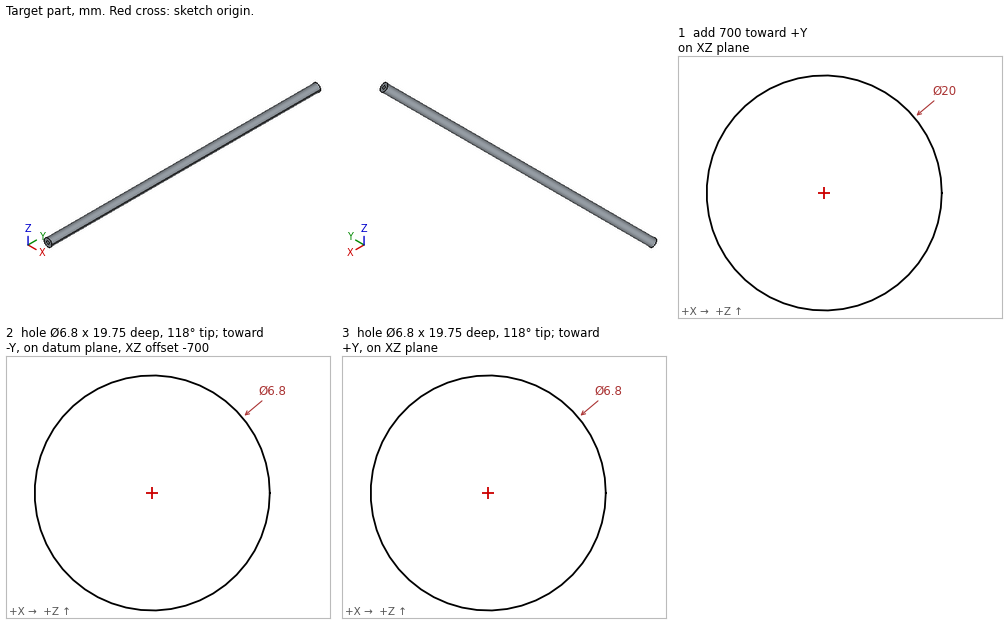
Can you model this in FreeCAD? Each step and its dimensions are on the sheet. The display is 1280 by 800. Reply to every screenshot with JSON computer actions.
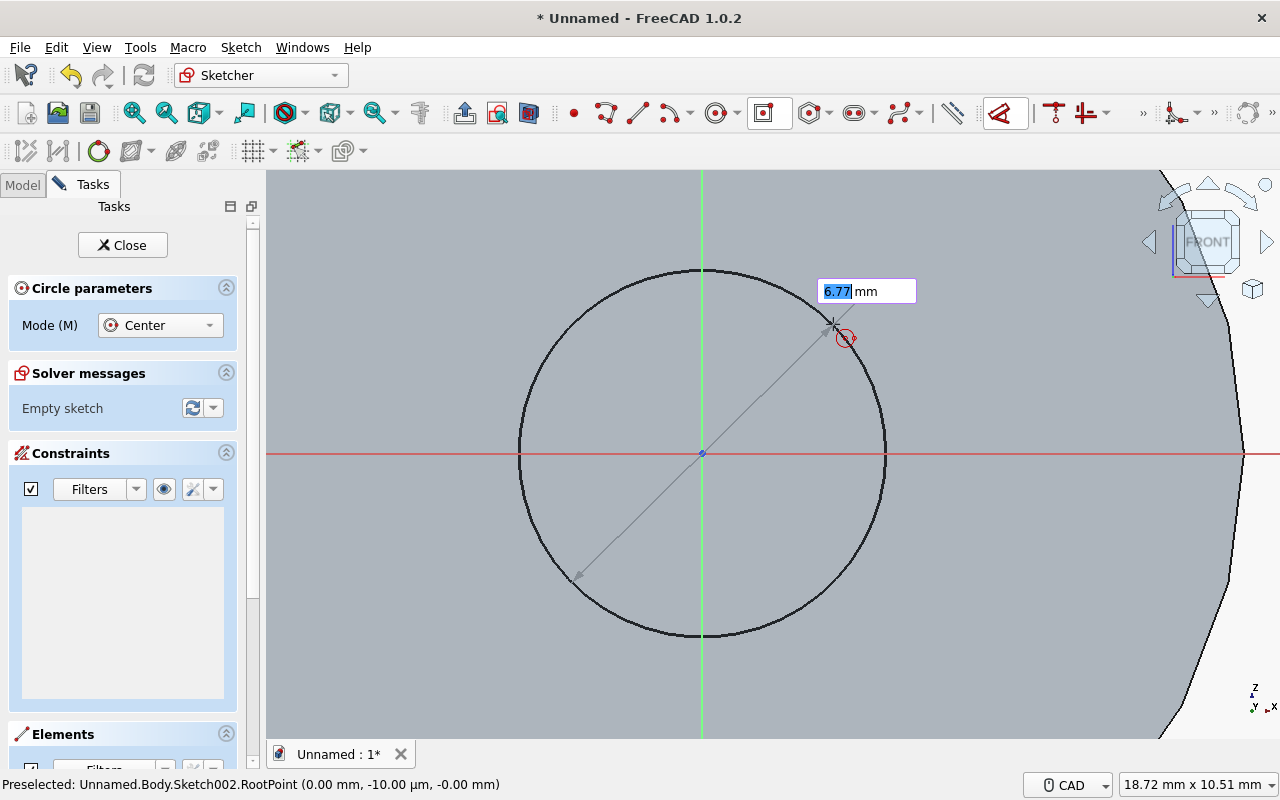
{"action": "type", "text": "6.8"}
{"action": "key", "text": "Return"}
{"action": "key", "text": "Escape"}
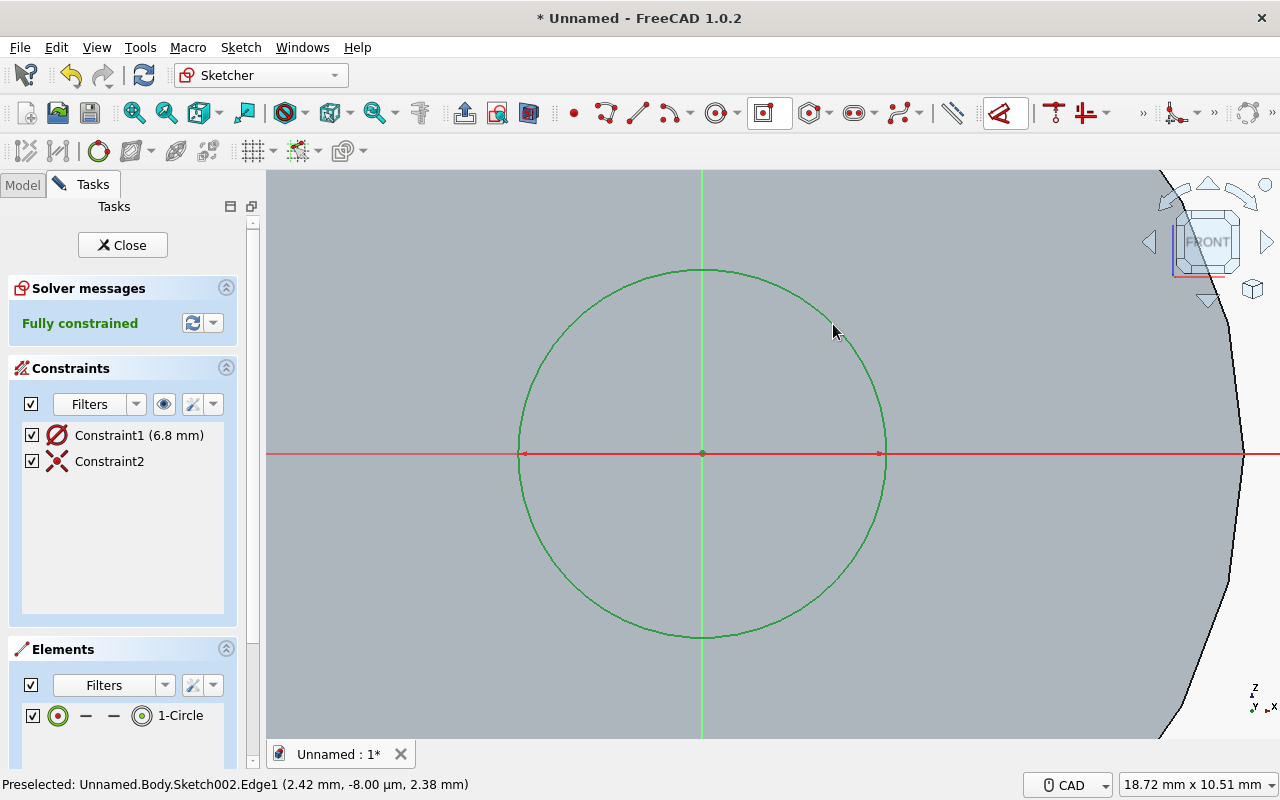
{"action": "left_click", "coordinate": [123, 245]}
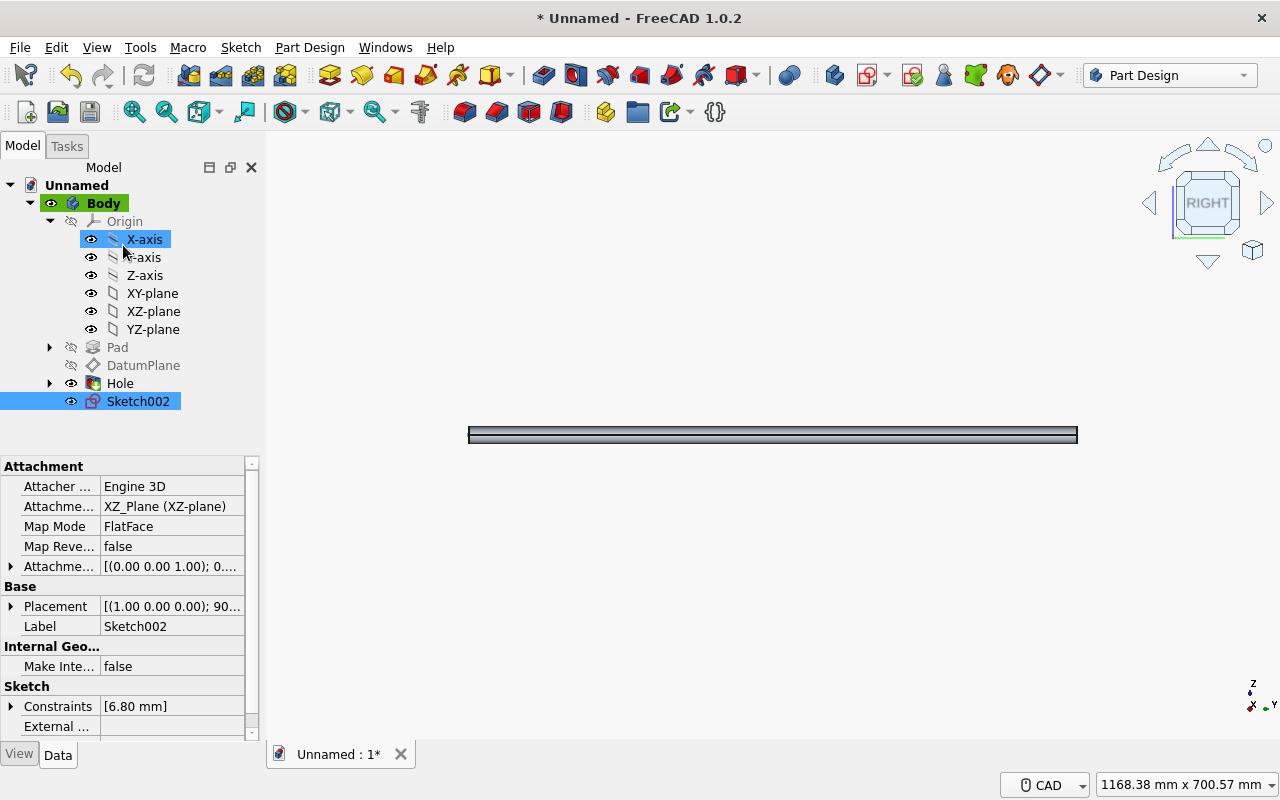
{"action": "left_click", "coordinate": [576, 76]}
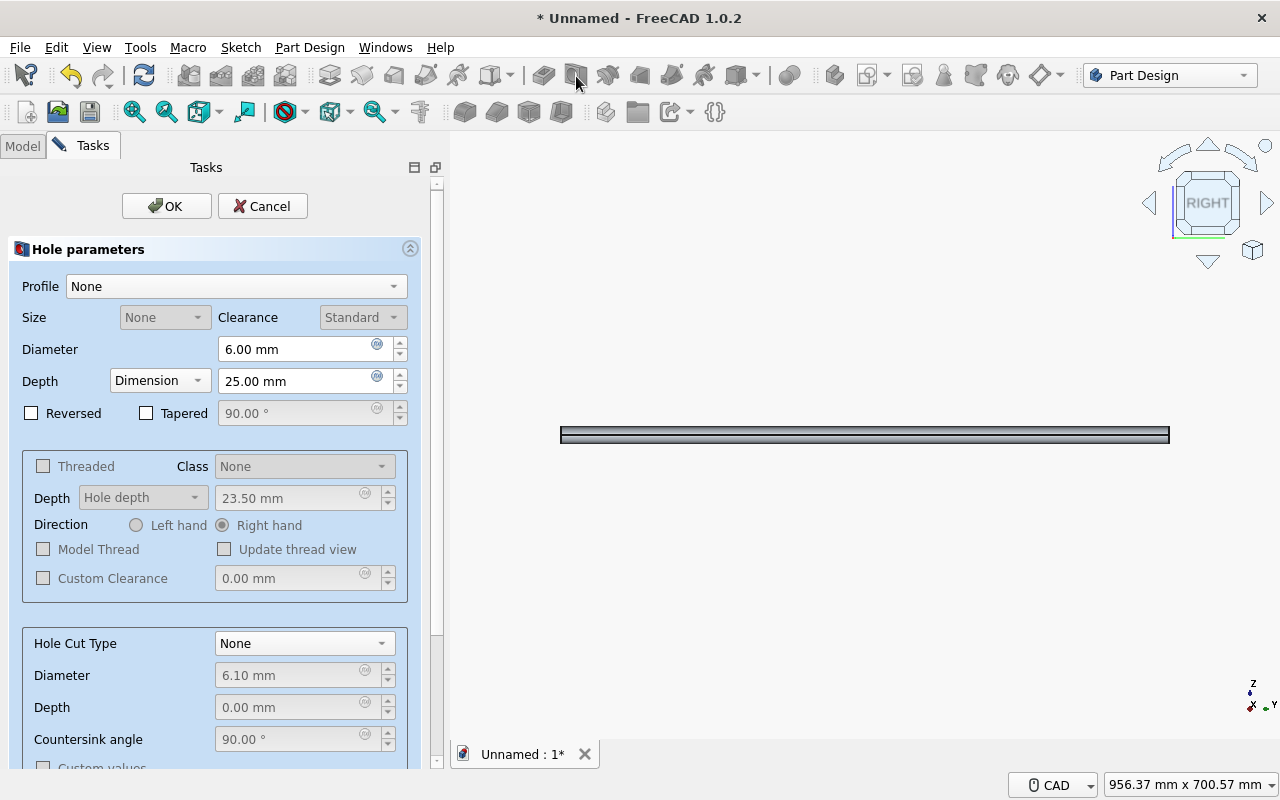
{"action": "triple_click", "coordinate": [305, 349]}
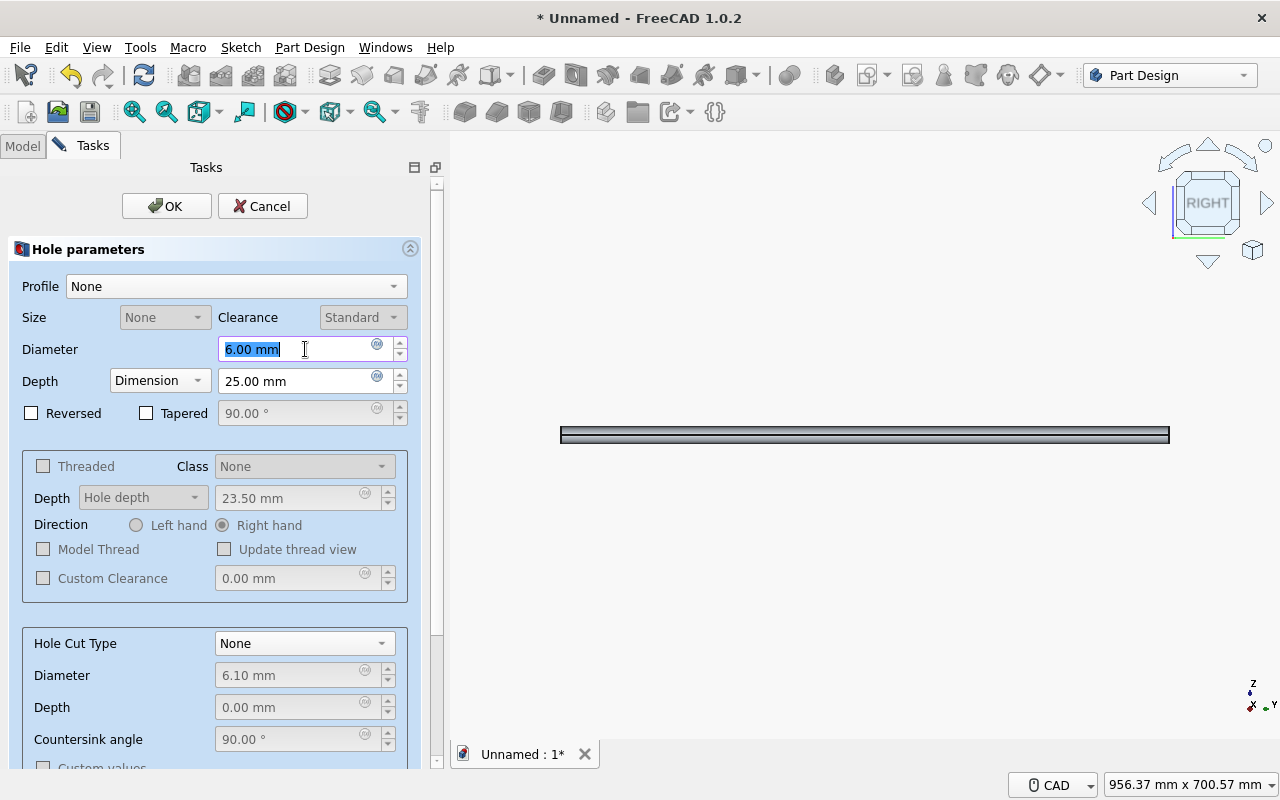
{"action": "type", "text": "6.8"}
{"action": "key", "text": "Tab"}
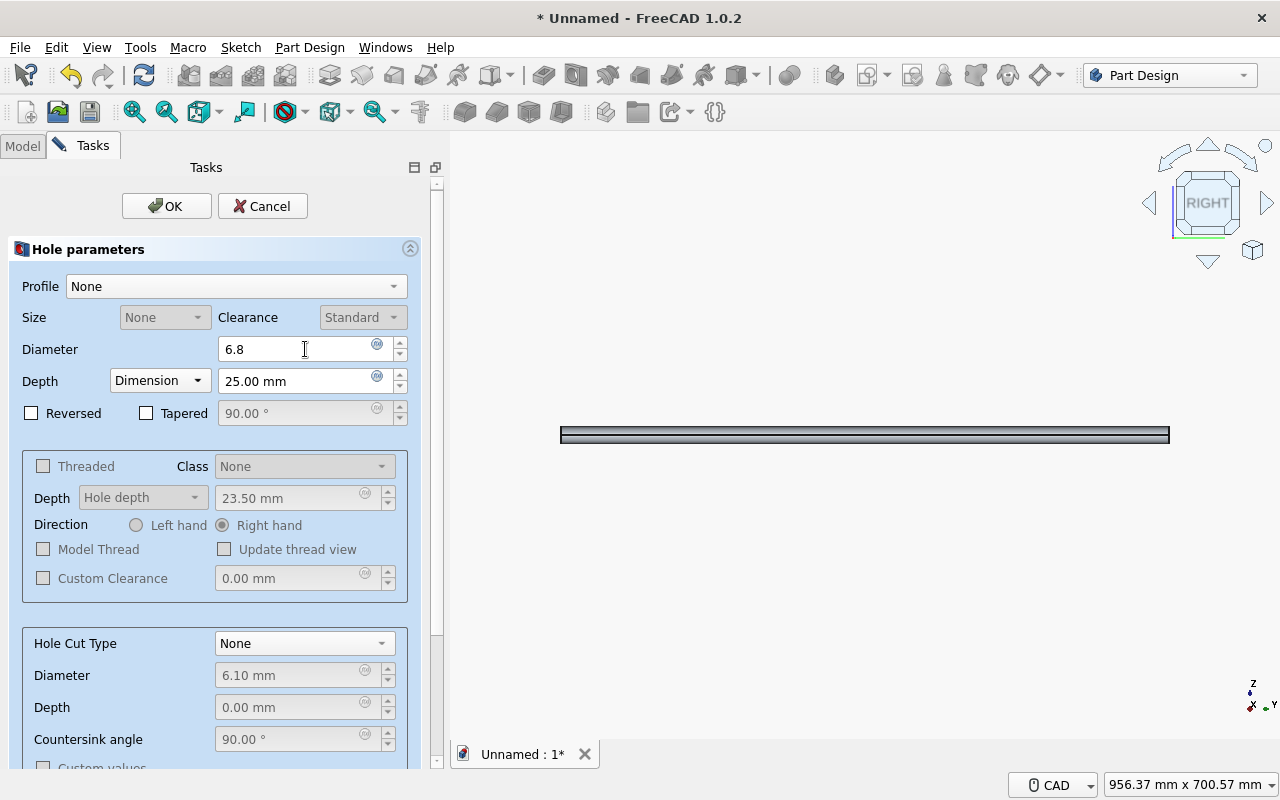
{"action": "triple_click", "coordinate": [305, 381]}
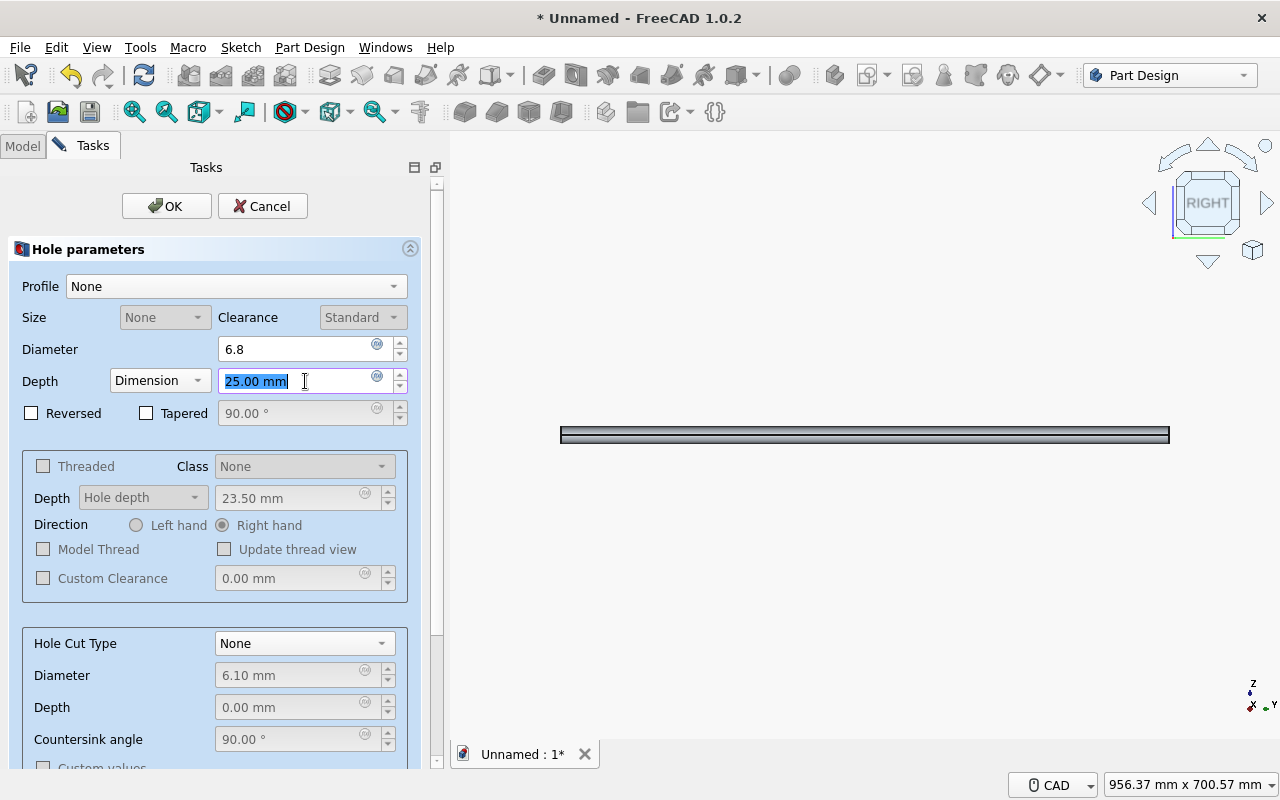
{"action": "type", "text": "19.75"}
{"action": "key", "text": "Tab"}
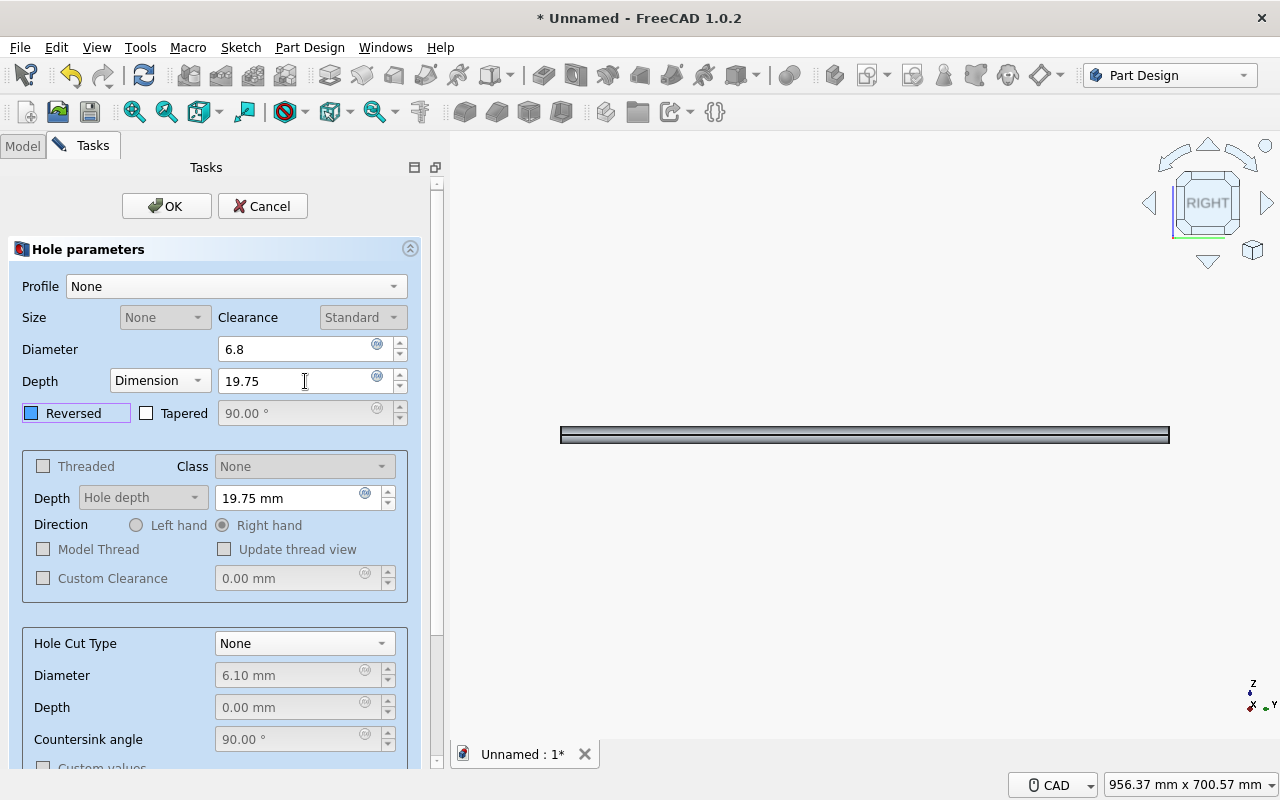
{"action": "left_click", "coordinate": [167, 206]}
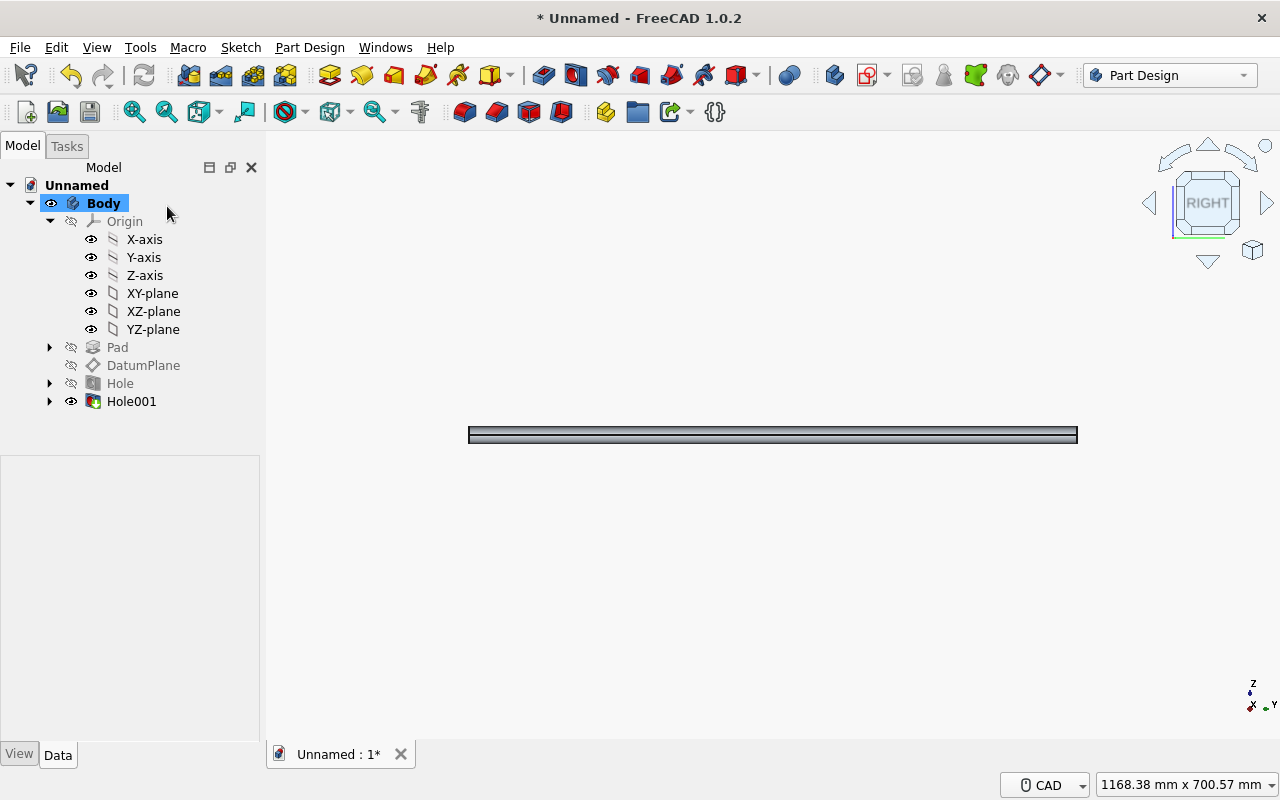
{"action": "key", "text": "0"}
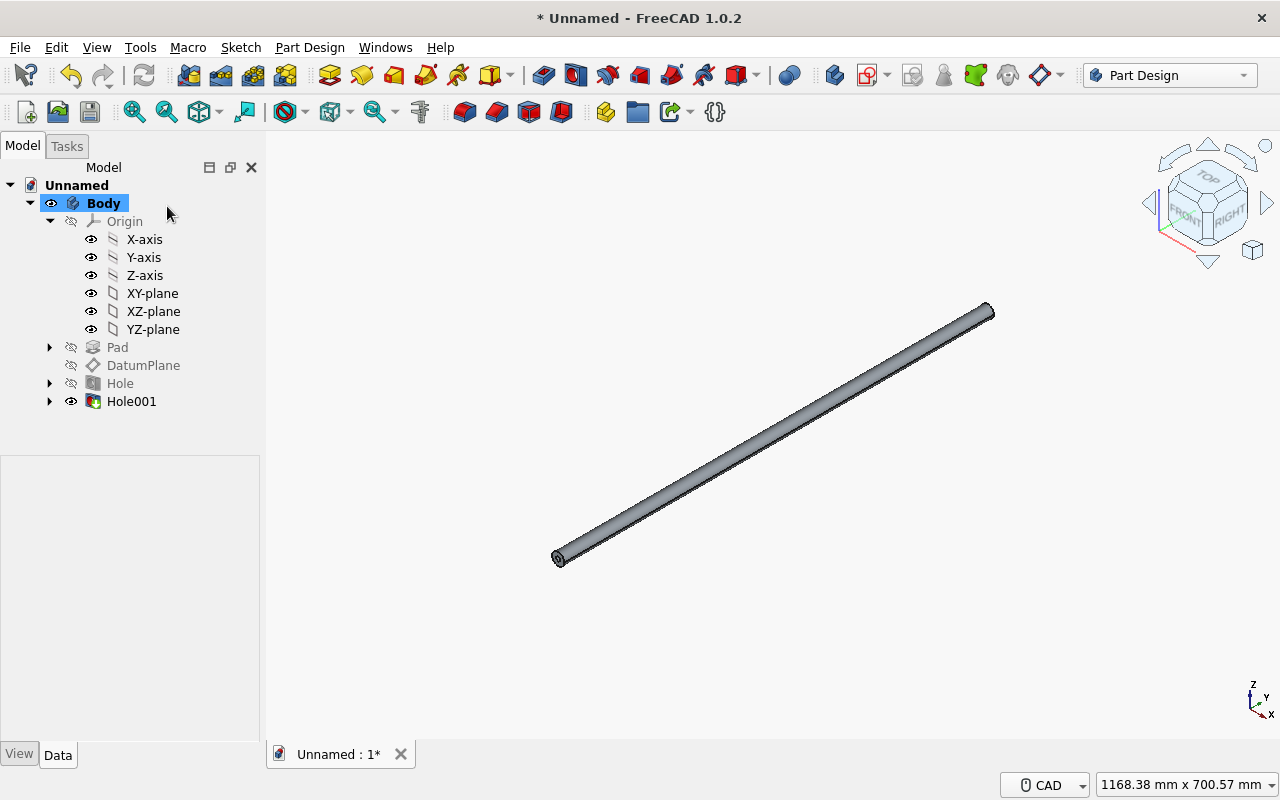
{"action": "left_click", "coordinate": [136, 112]}